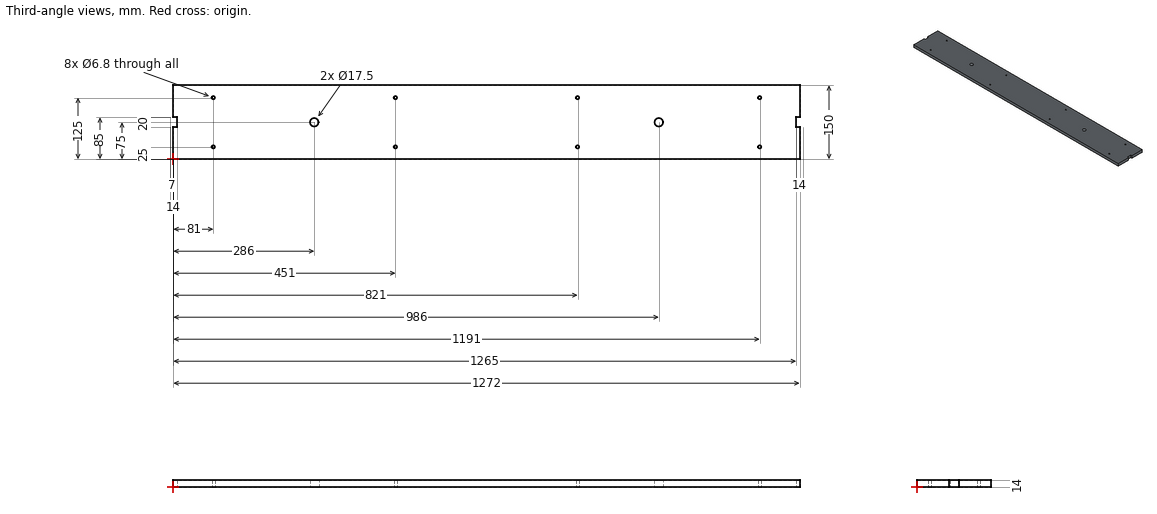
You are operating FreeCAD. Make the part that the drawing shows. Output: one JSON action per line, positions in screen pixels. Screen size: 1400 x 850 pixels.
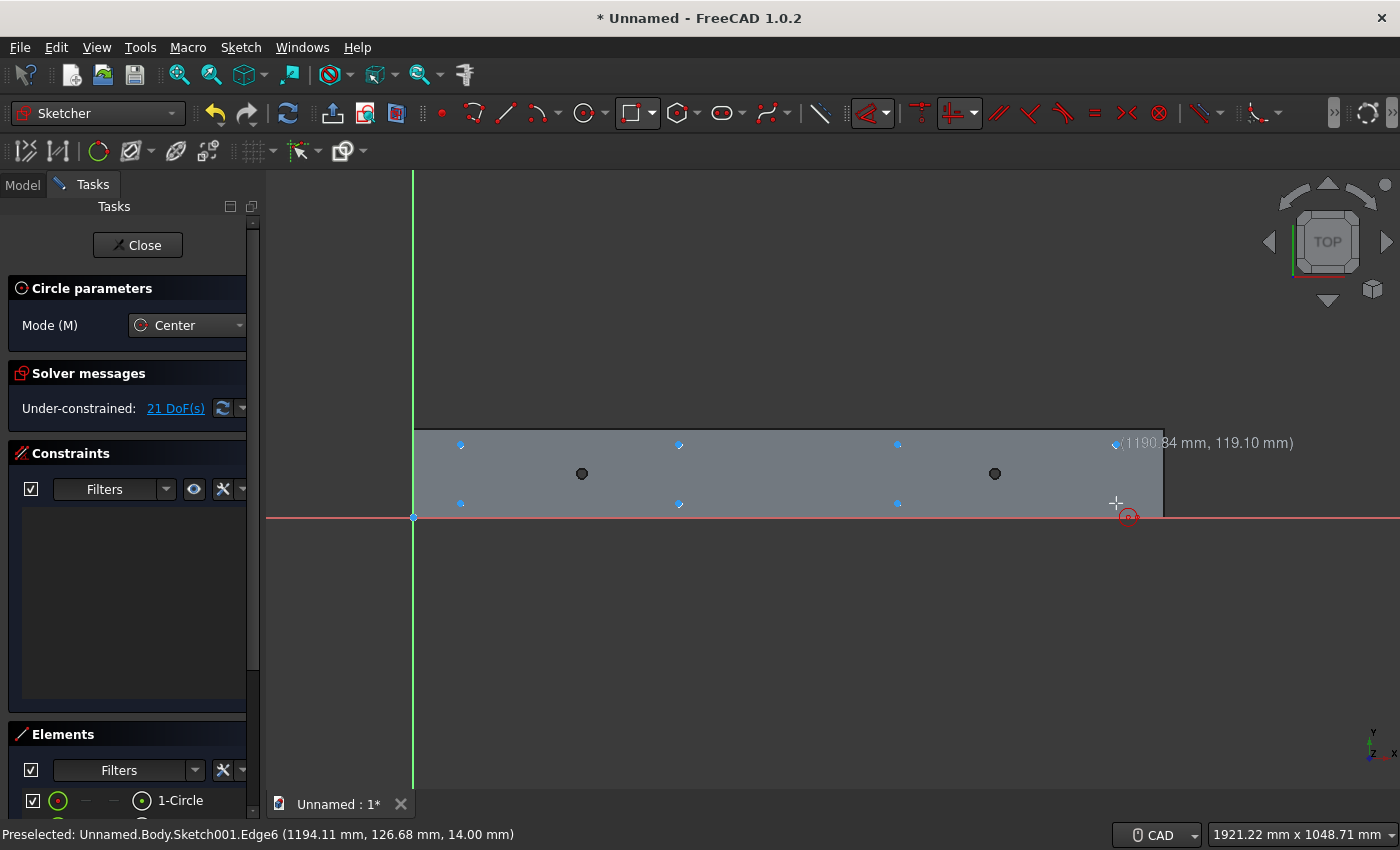
{"action": "left_click", "coordinate": [1116, 503]}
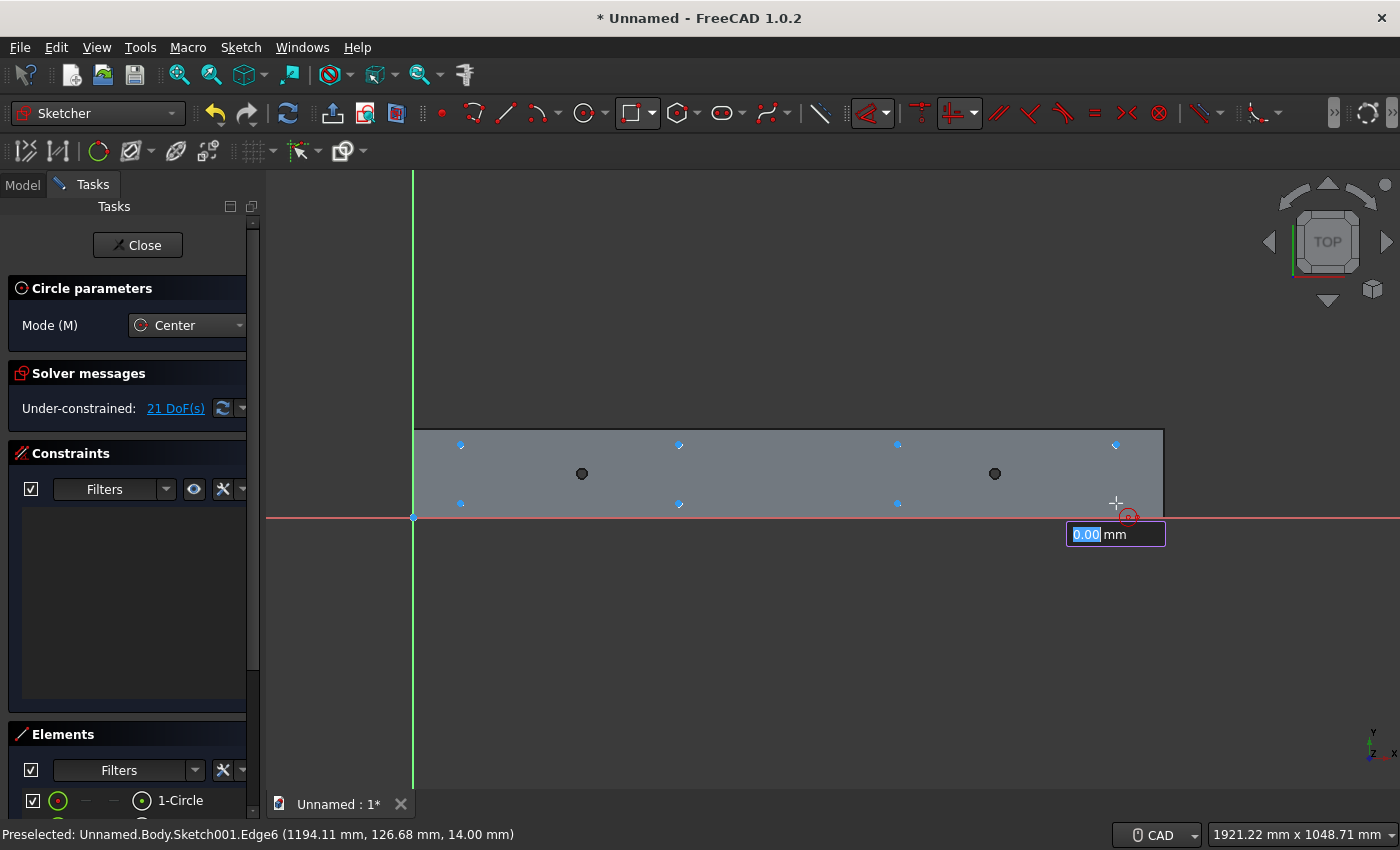
{"action": "scroll", "coordinate": [1118, 502], "scroll_direction": "up", "scroll_amount": 11}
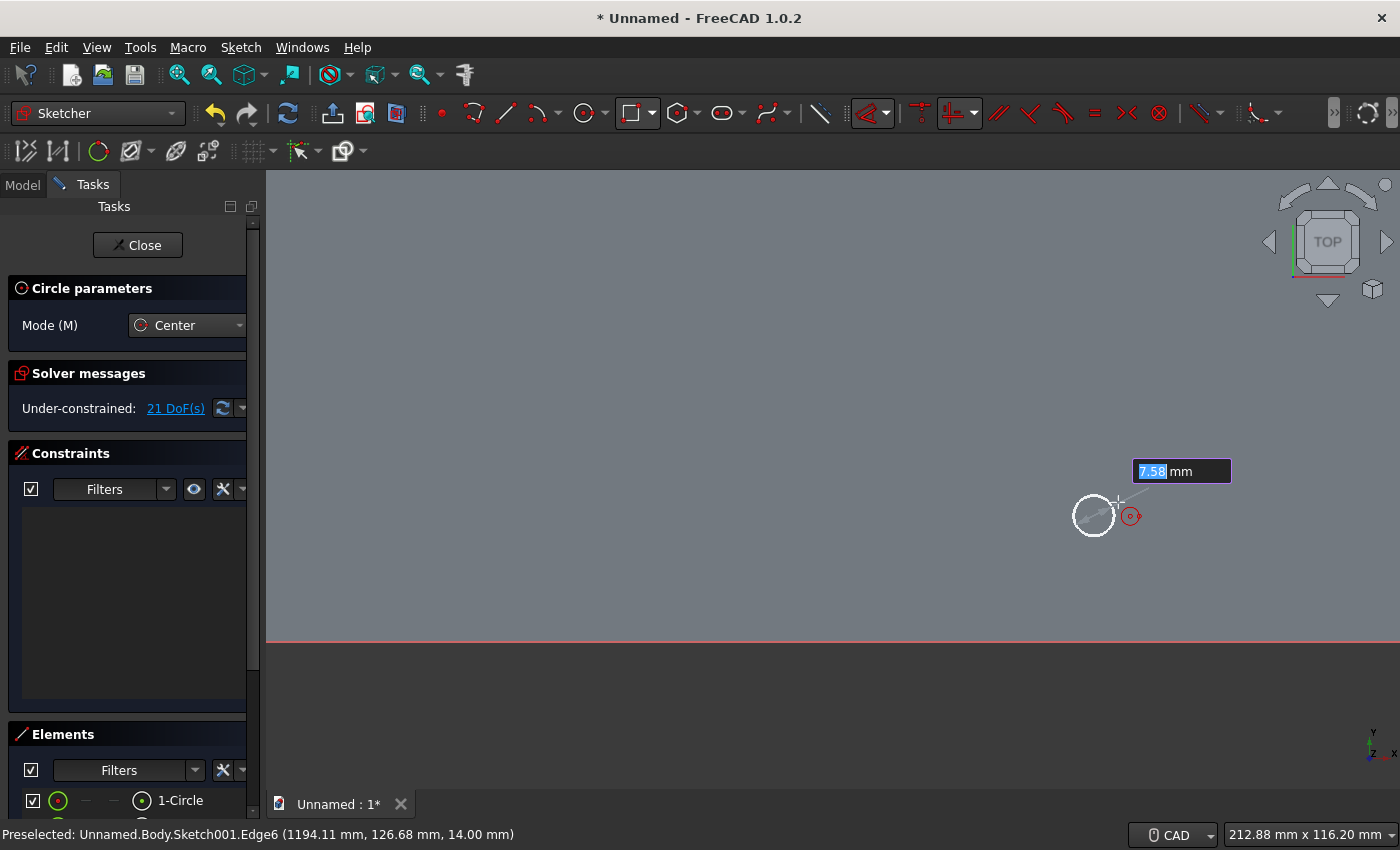
{"action": "left_click", "coordinate": [1108, 496]}
{"action": "key", "text": "Escape"}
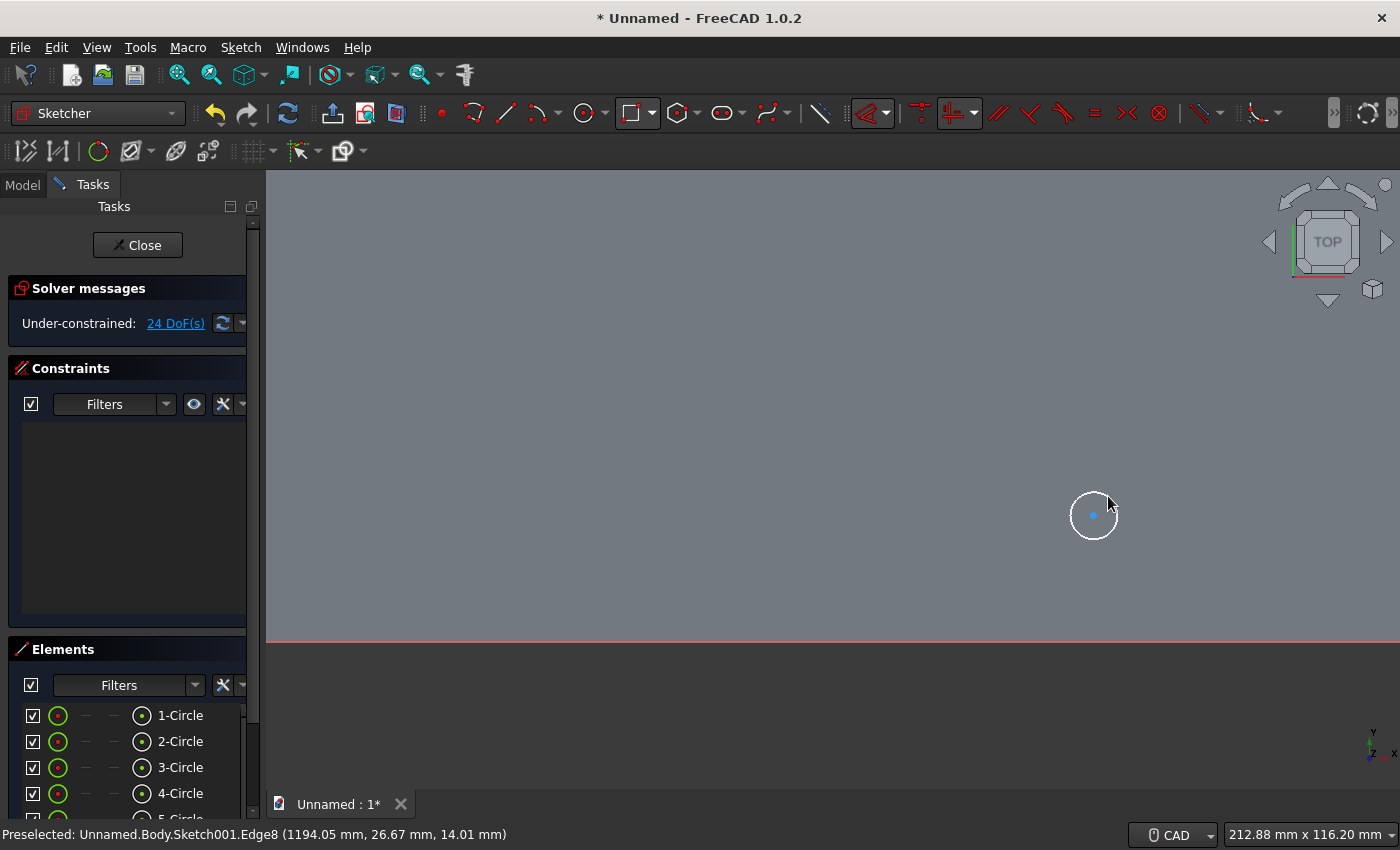
{"action": "scroll", "coordinate": [1118, 502], "scroll_direction": "down", "scroll_amount": 11}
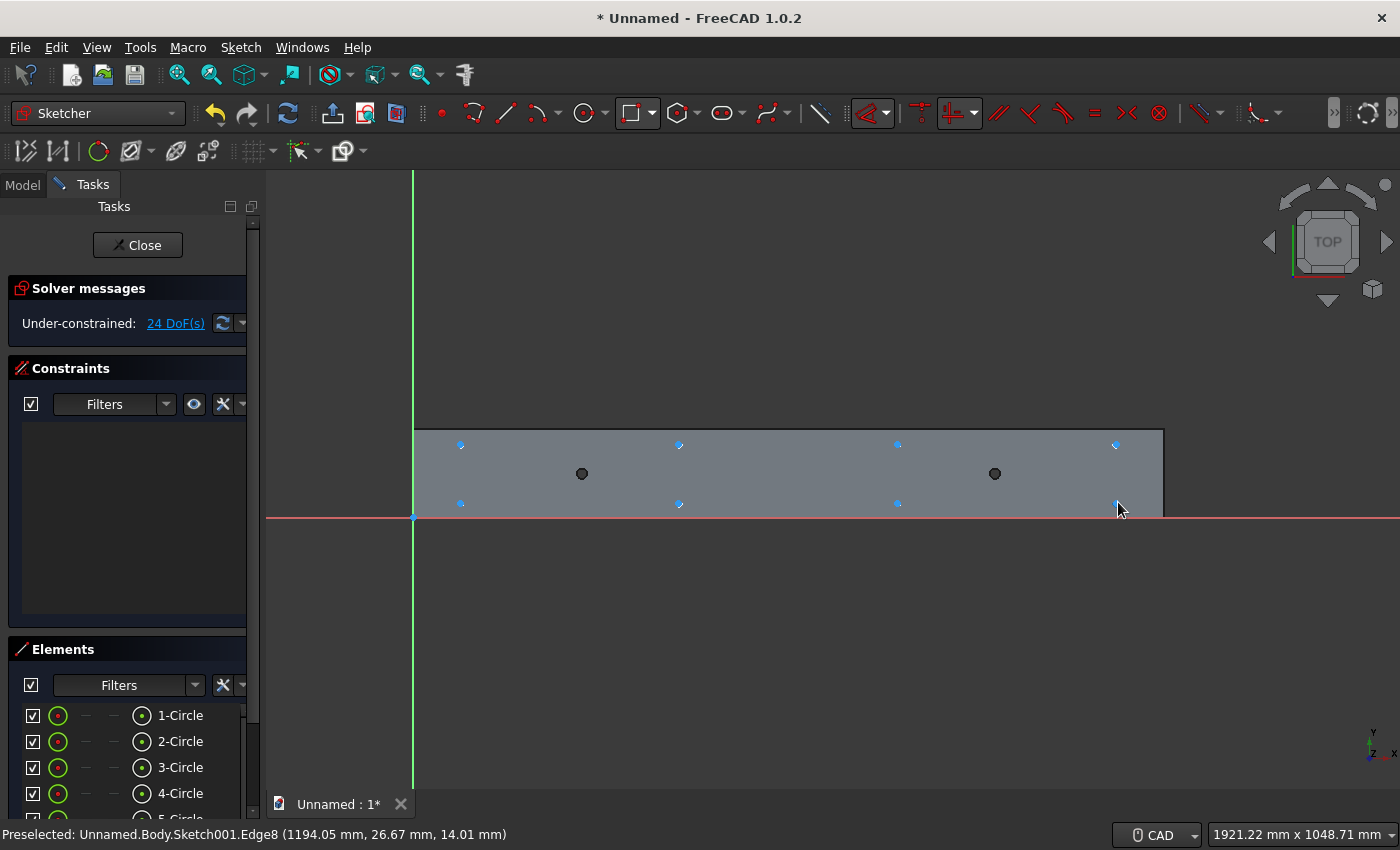
{"action": "scroll", "coordinate": [463, 443], "scroll_direction": "up", "scroll_amount": 9}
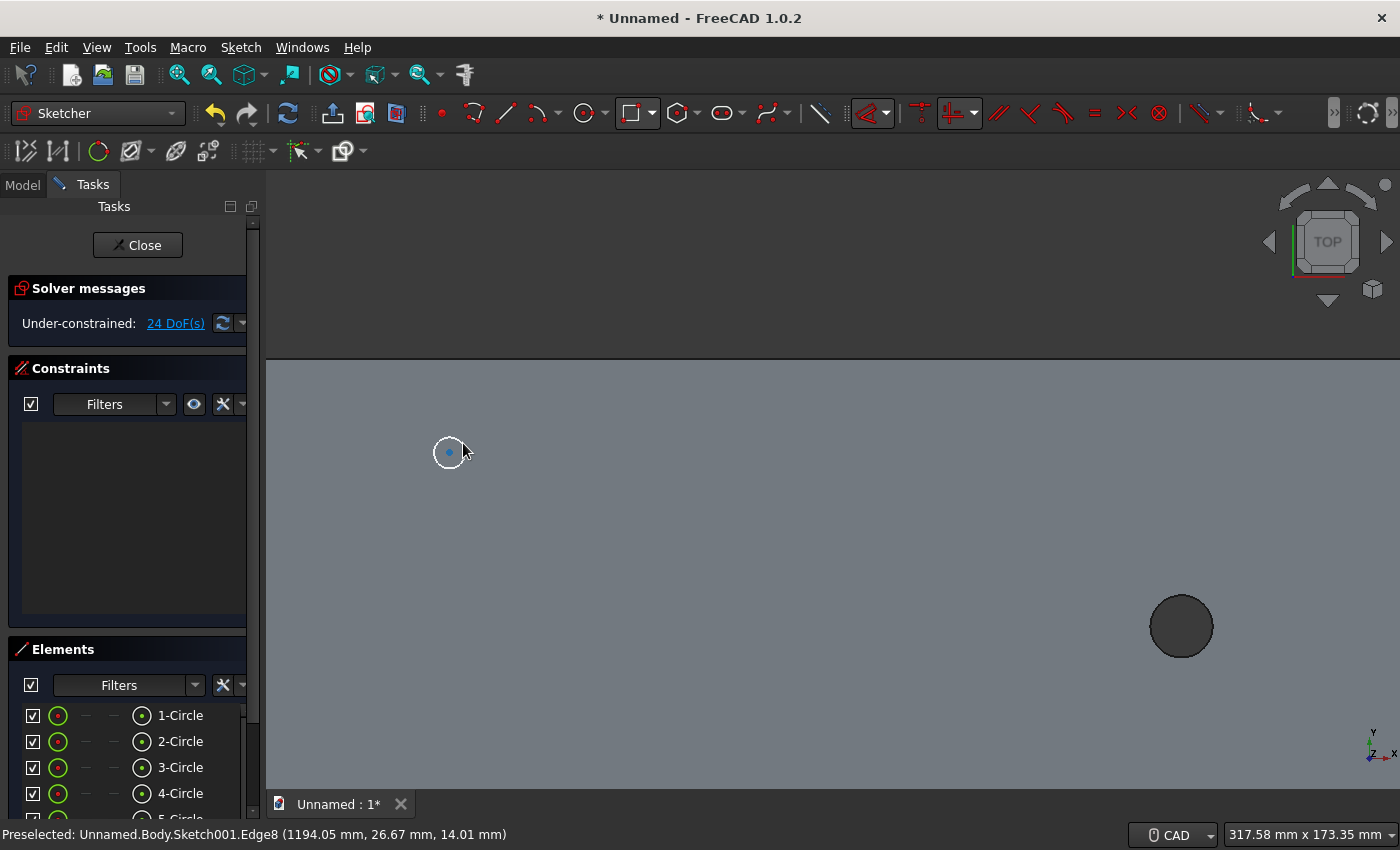
{"action": "left_click", "coordinate": [461, 442]}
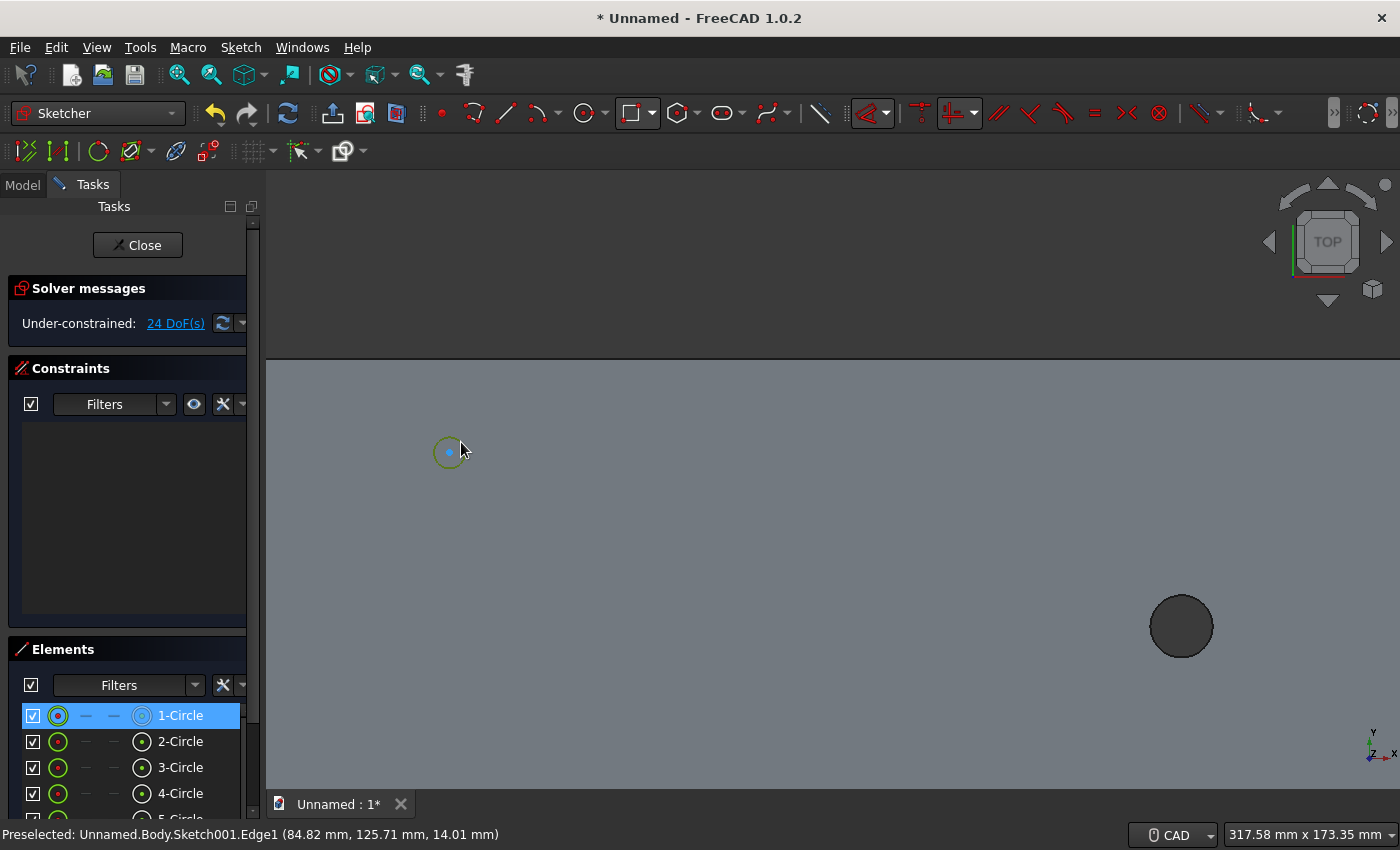
{"action": "scroll", "coordinate": [462, 443], "scroll_direction": "down", "scroll_amount": 9}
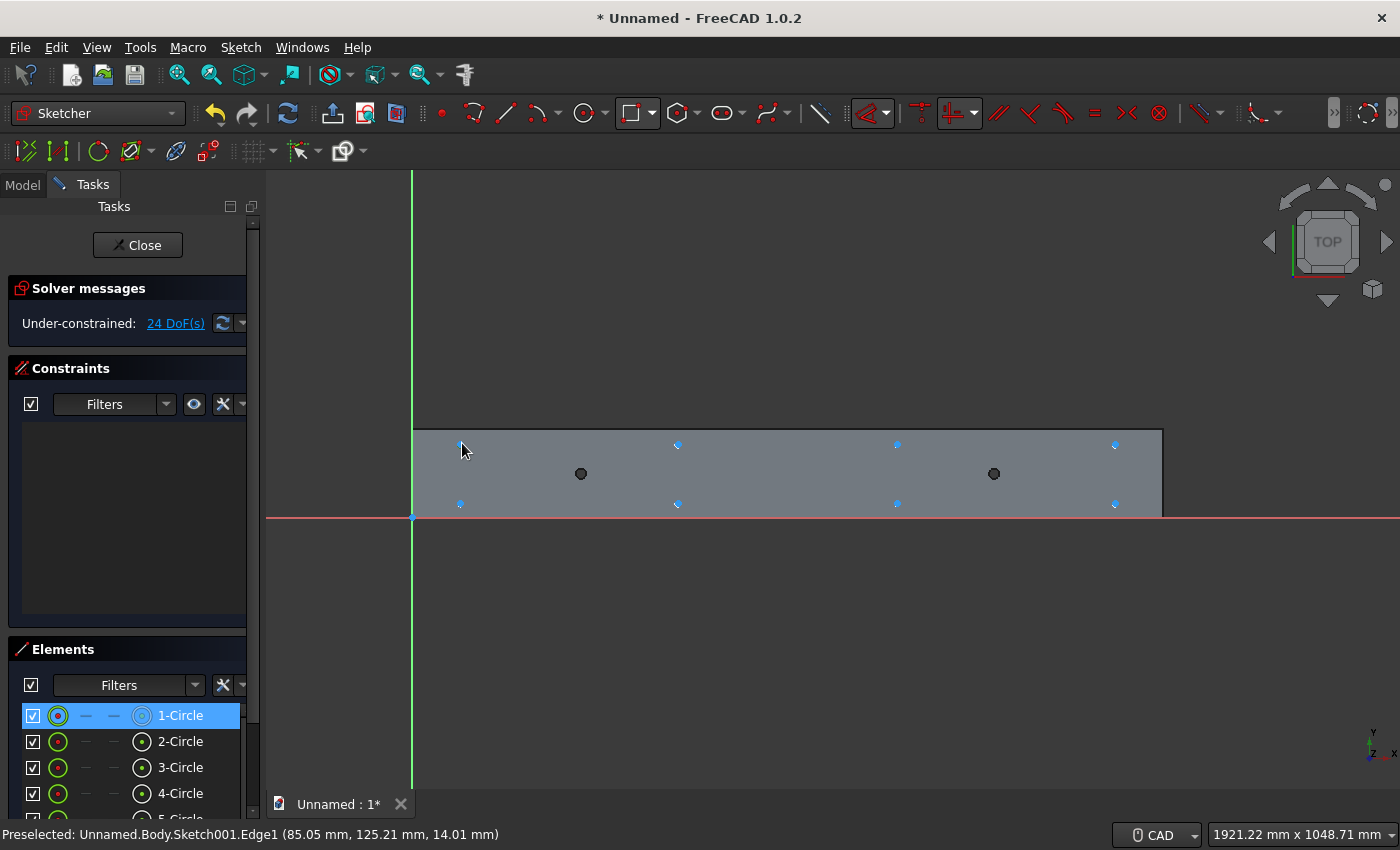
{"action": "scroll", "coordinate": [462, 502], "scroll_direction": "up", "scroll_amount": 9}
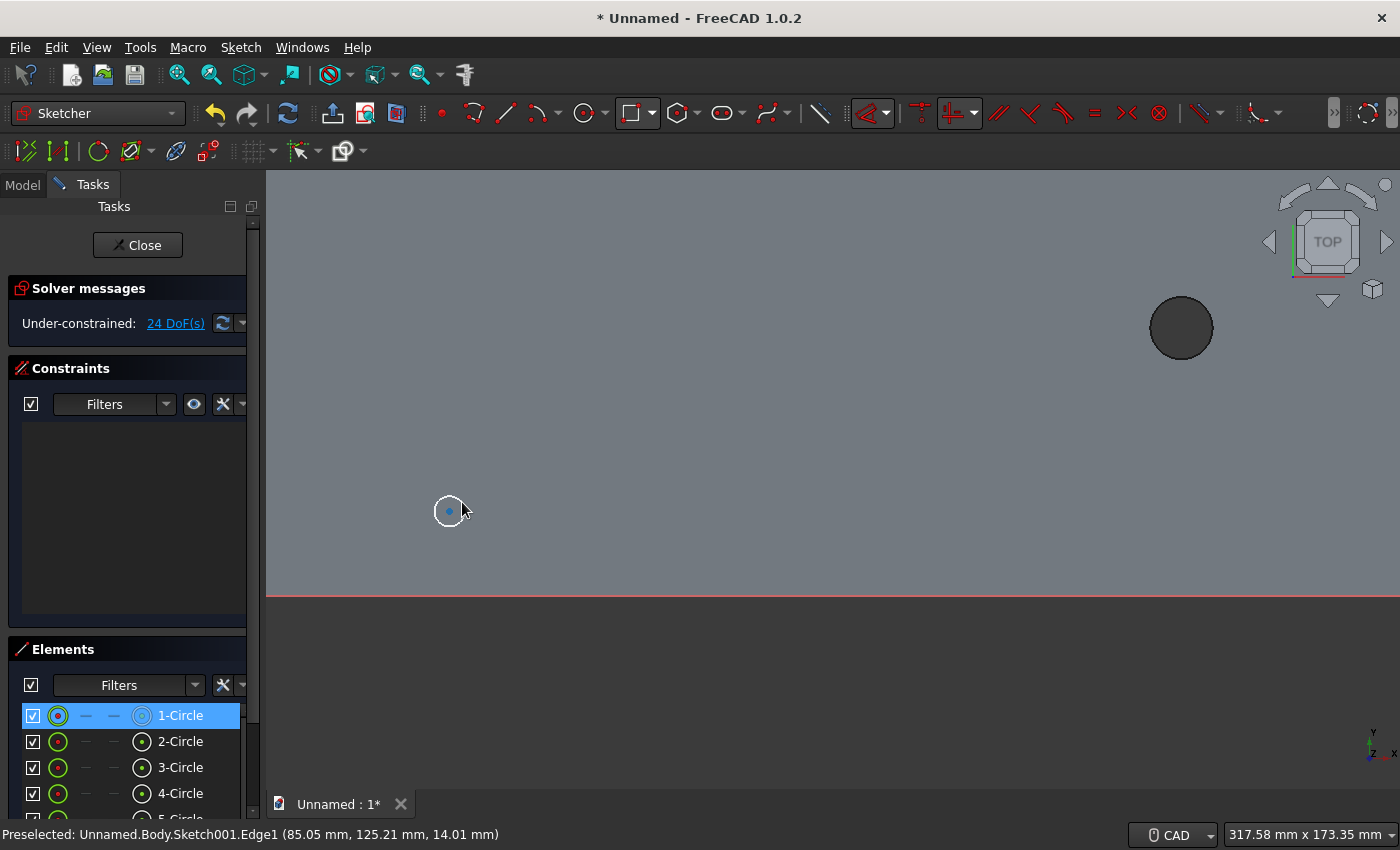
{"action": "left_click", "coordinate": [460, 501]}